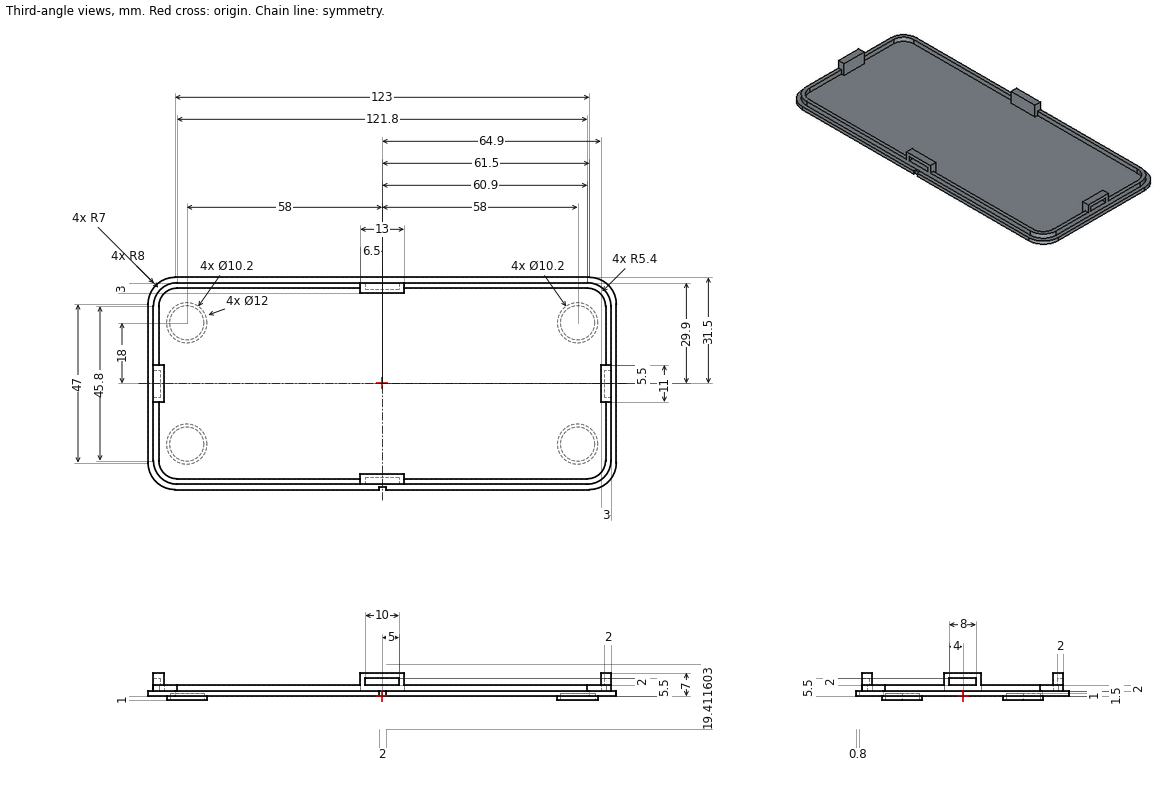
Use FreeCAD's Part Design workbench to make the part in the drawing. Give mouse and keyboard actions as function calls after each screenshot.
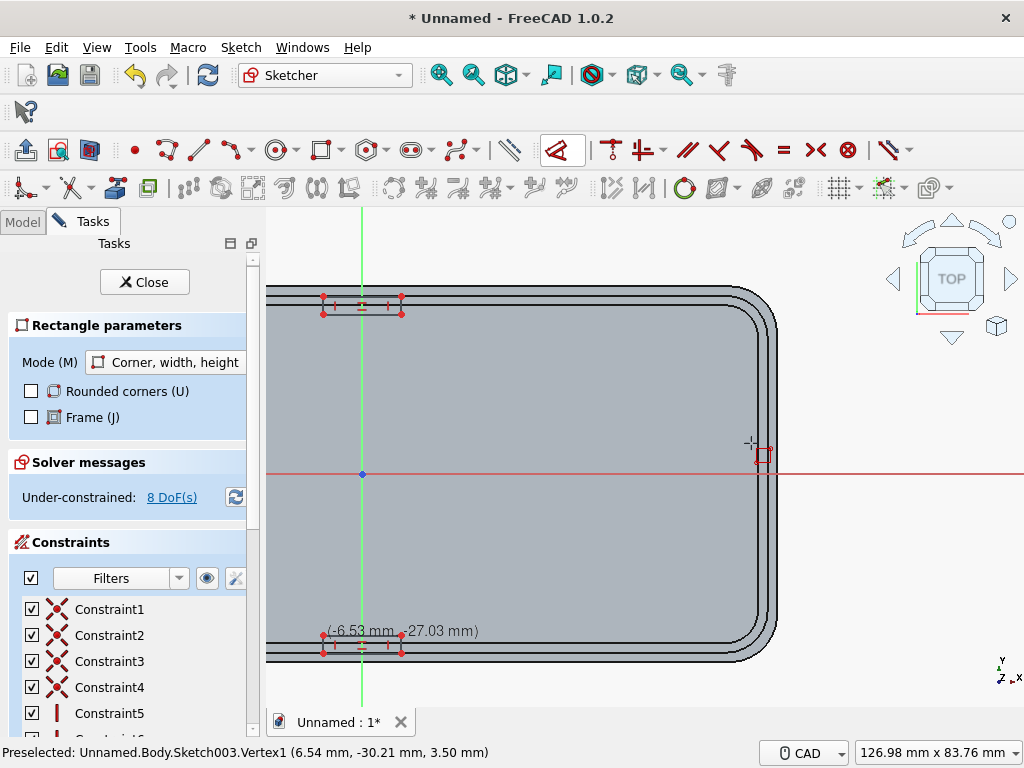
click(750, 441)
click(768, 507)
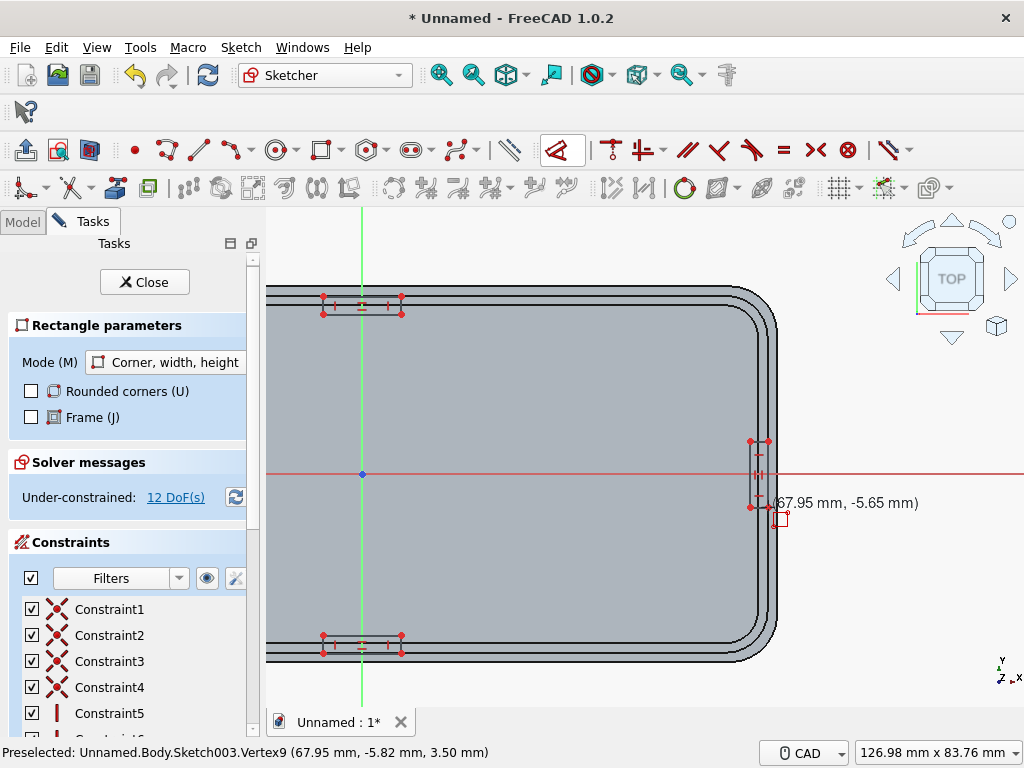
scroll(751, 443, down, 4)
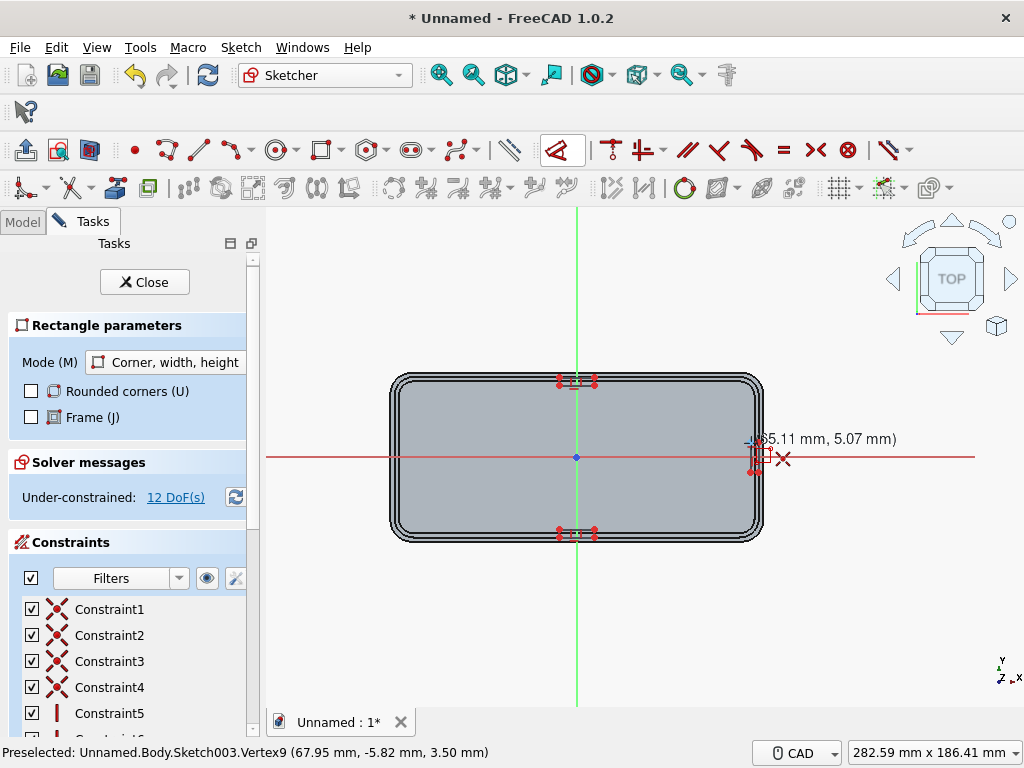
scroll(395, 443, up, 4)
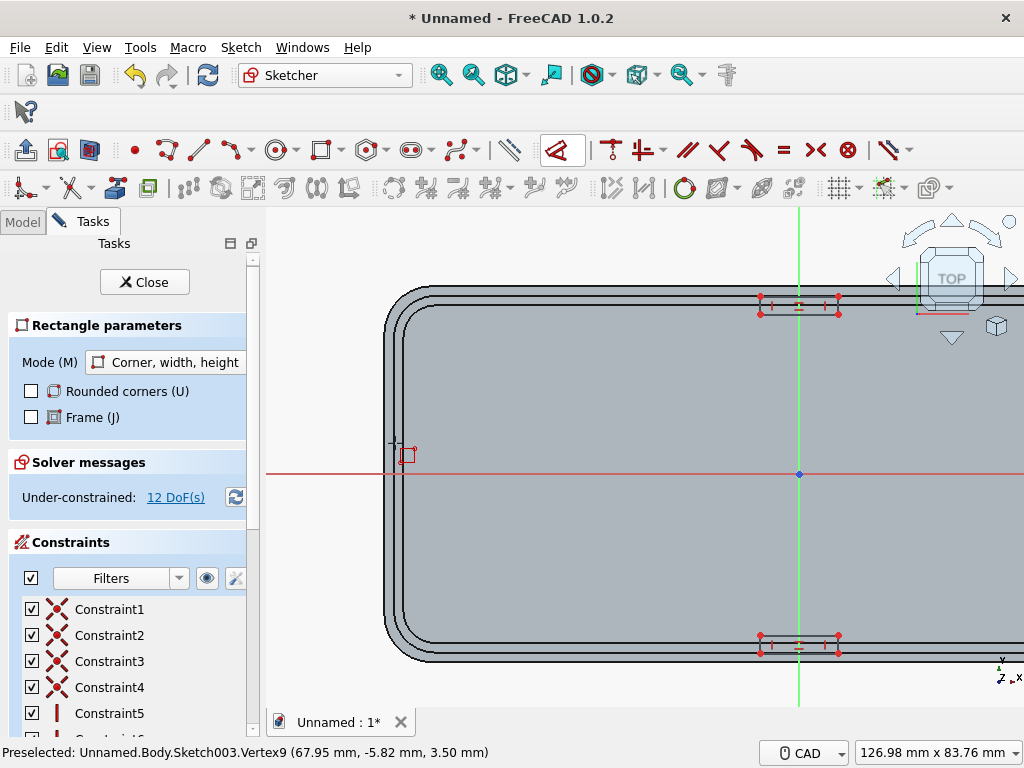
click(394, 441)
click(412, 507)
key(Escape)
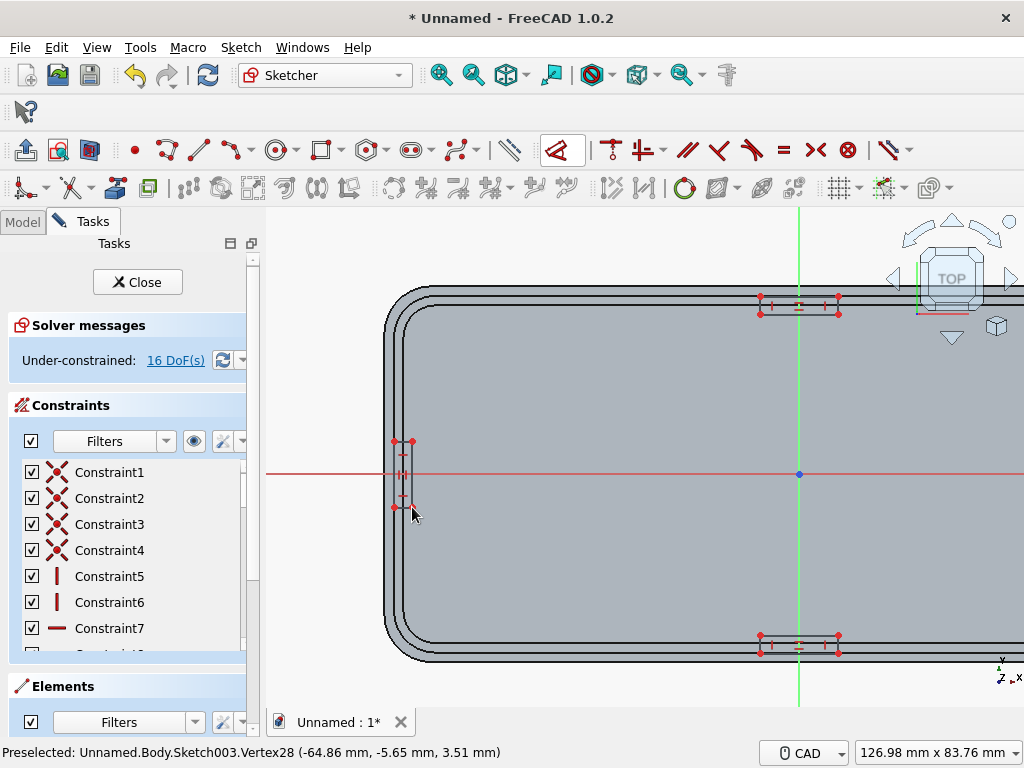
click(760, 315)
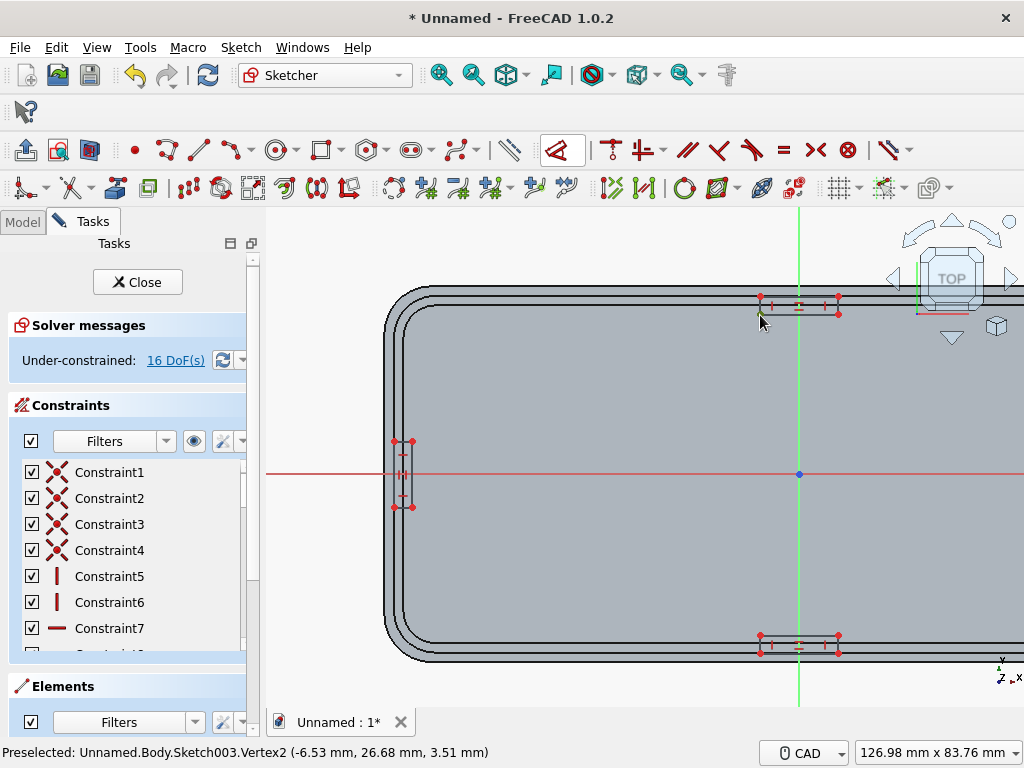
click(760, 636)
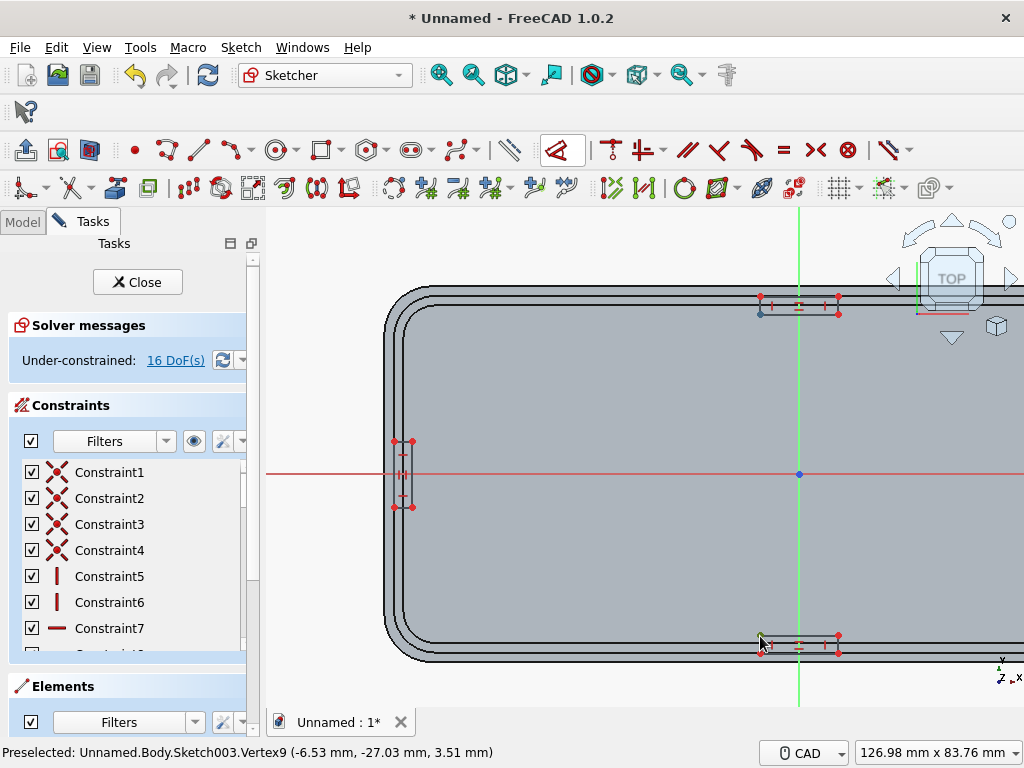
click(334, 474)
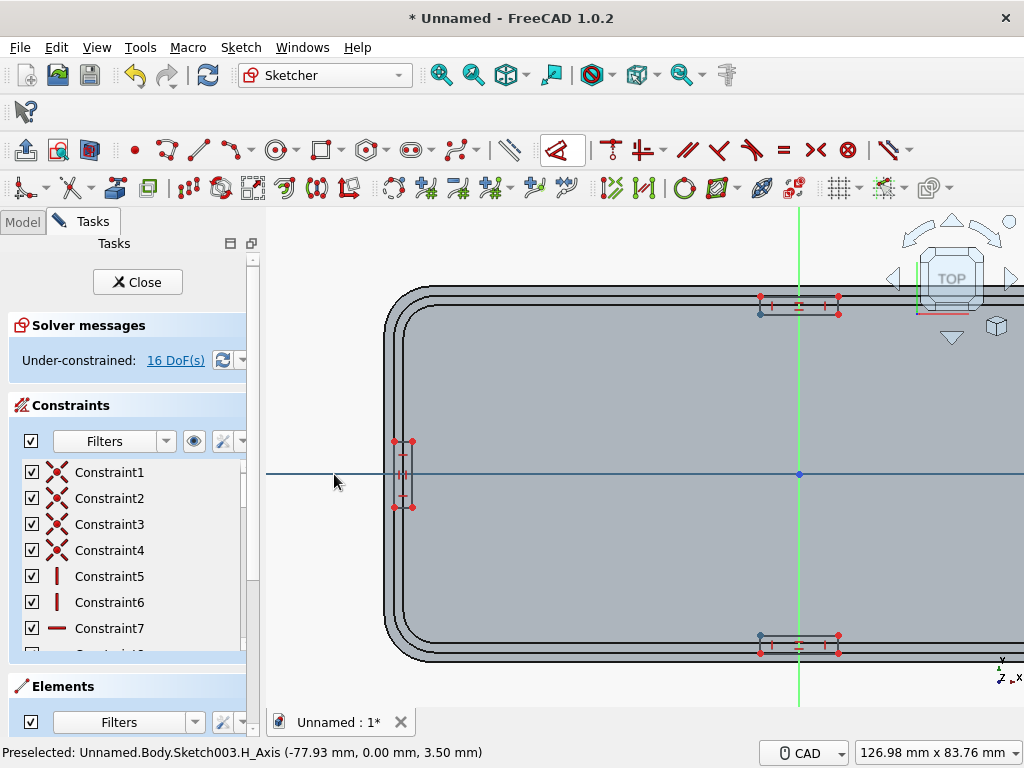
click(816, 150)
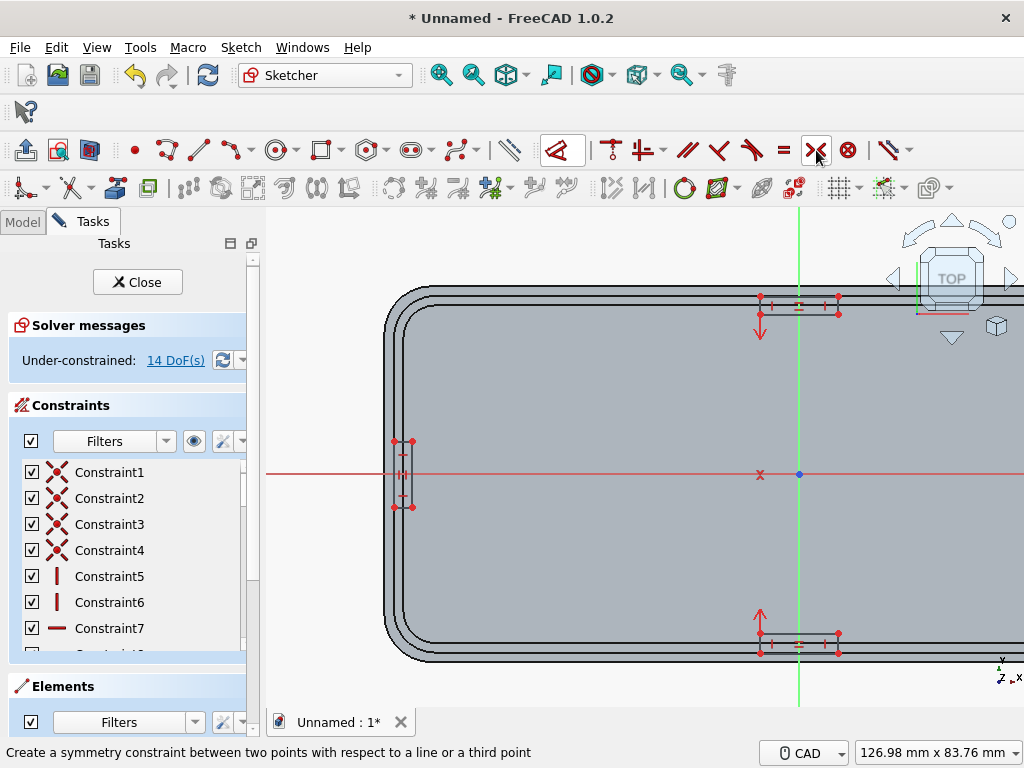
click(838, 297)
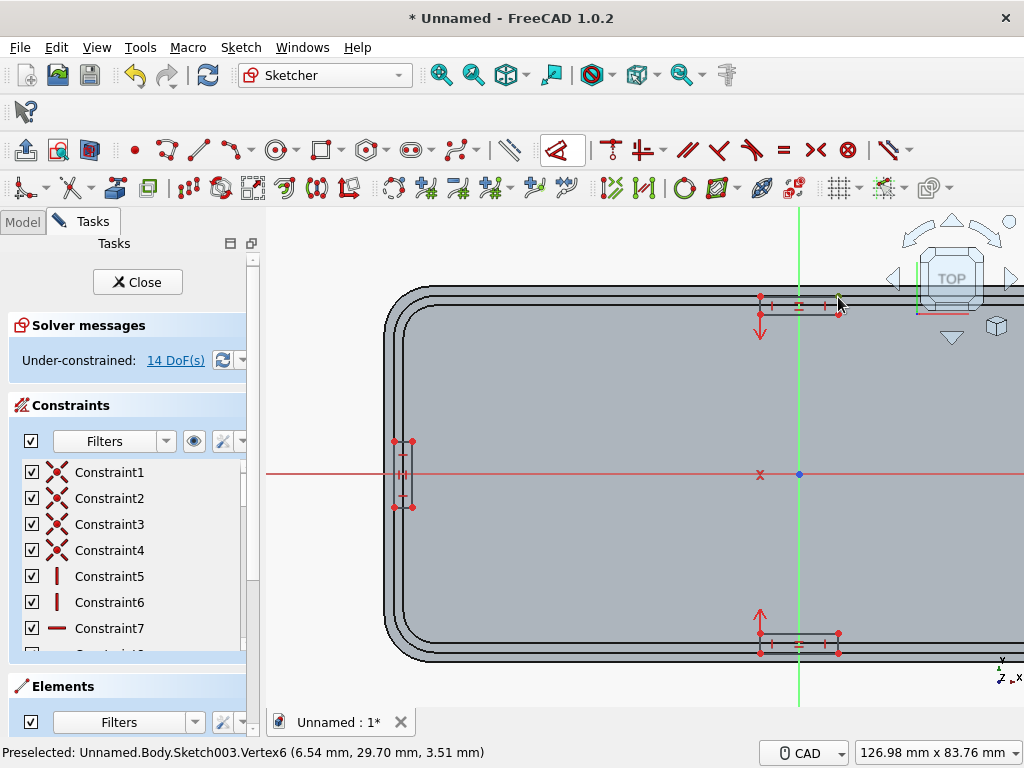
click(838, 654)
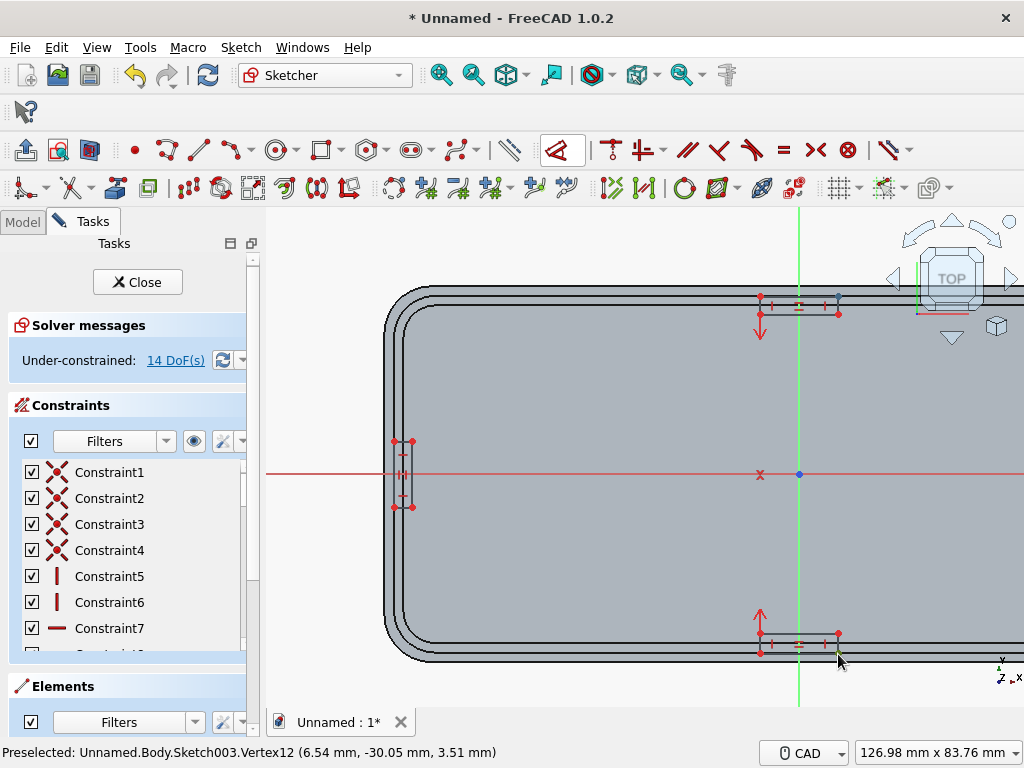
click(334, 474)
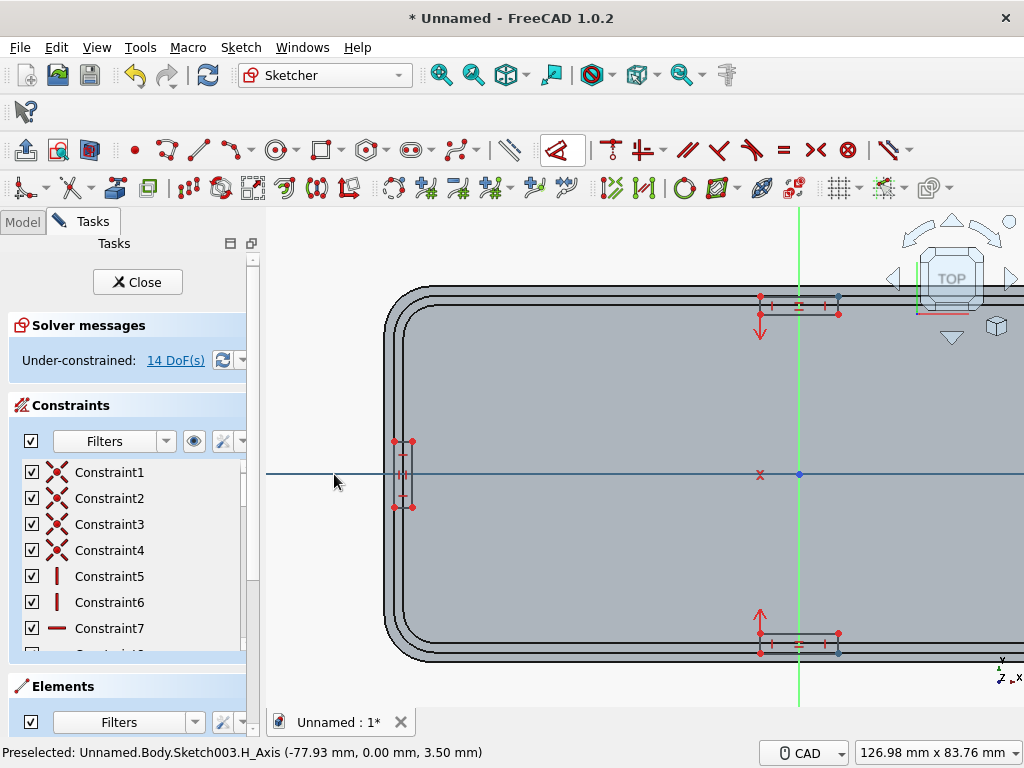
click(816, 150)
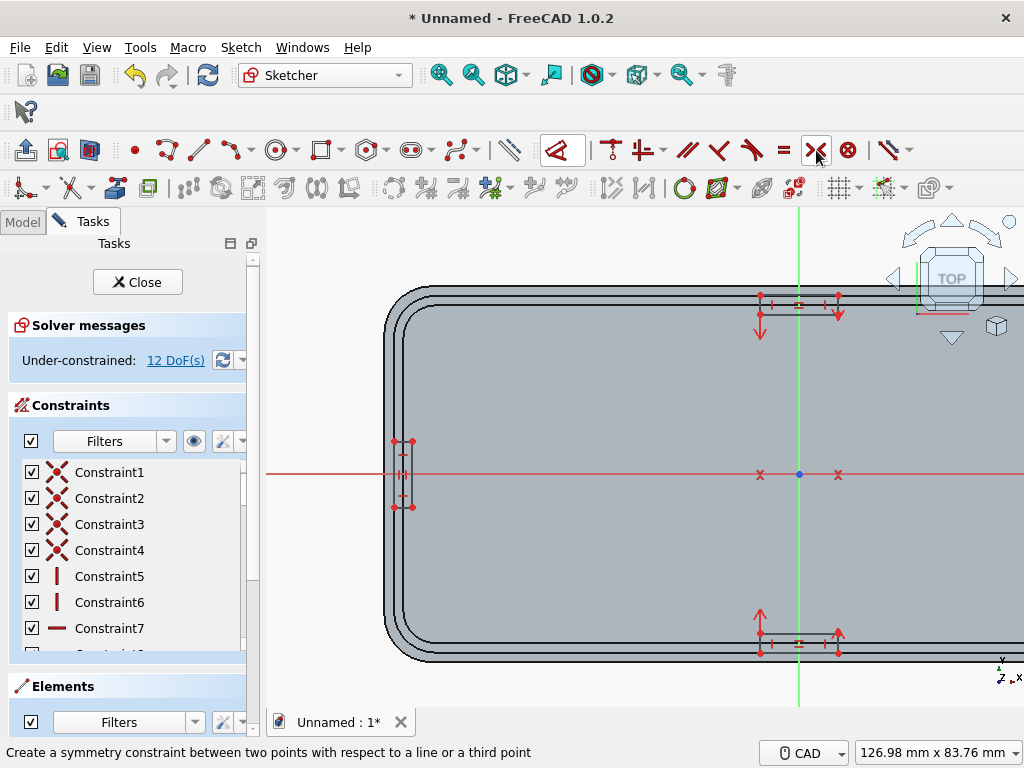
scroll(395, 443, down, 4)